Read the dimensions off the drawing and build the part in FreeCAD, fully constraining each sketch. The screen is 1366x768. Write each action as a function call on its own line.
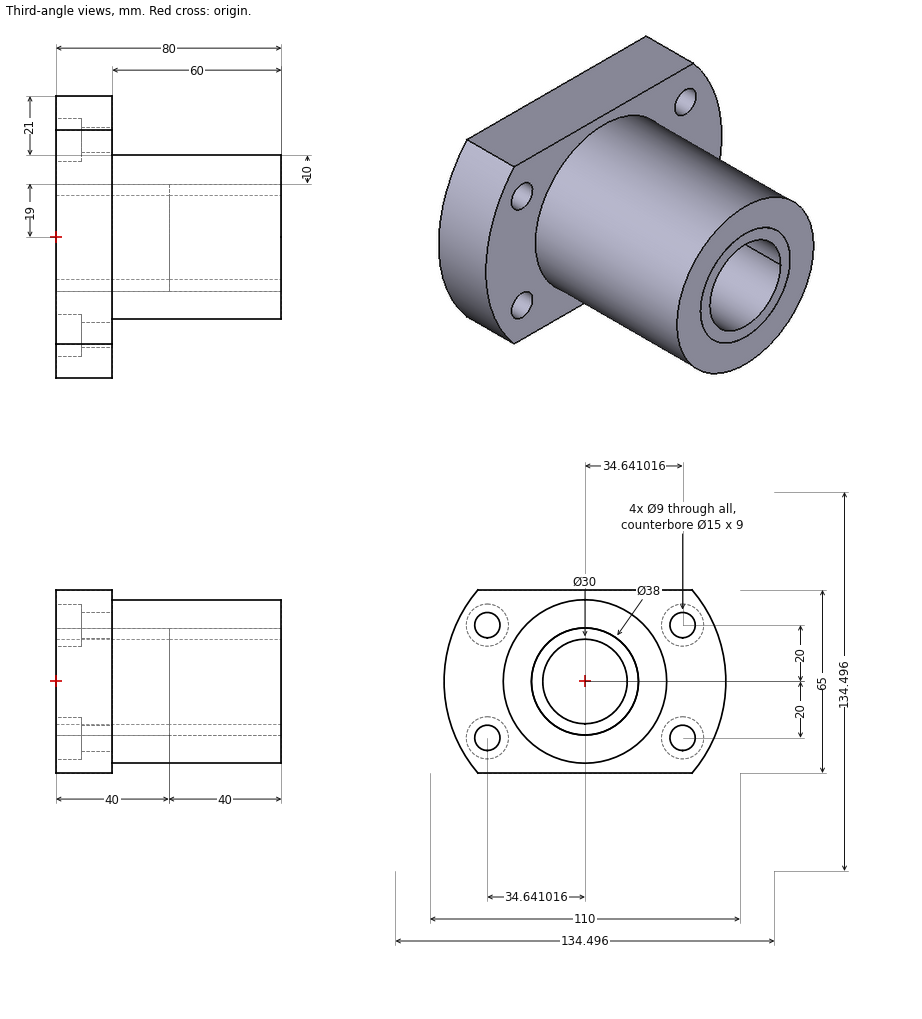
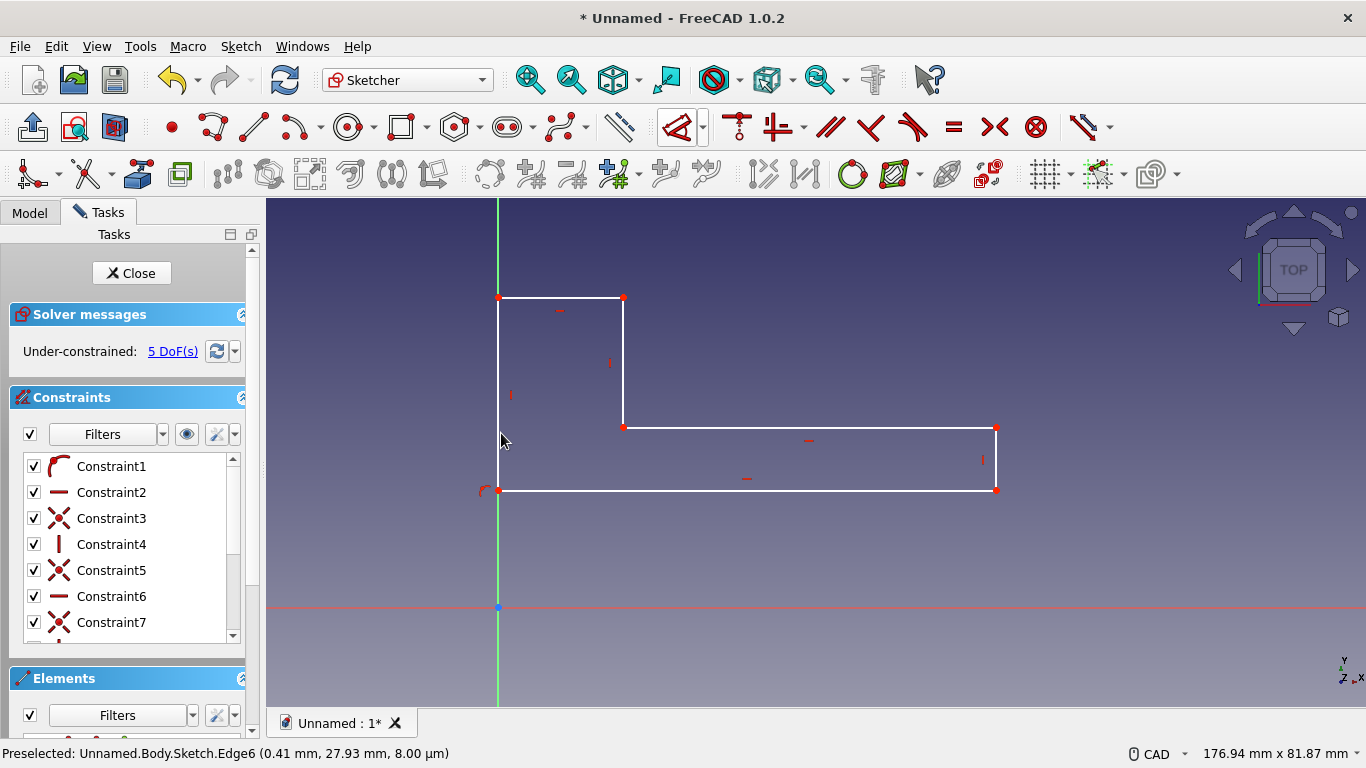
key(d)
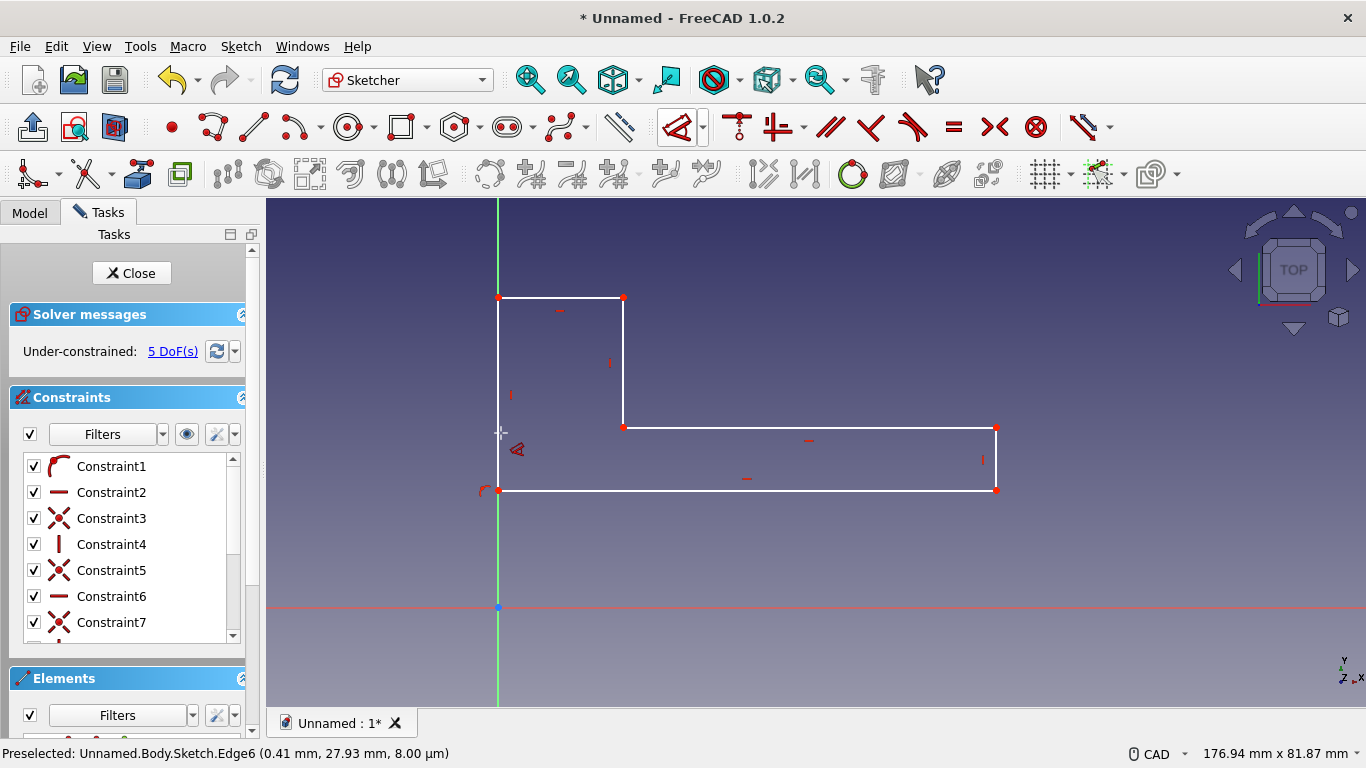
click(648, 491)
click(747, 525)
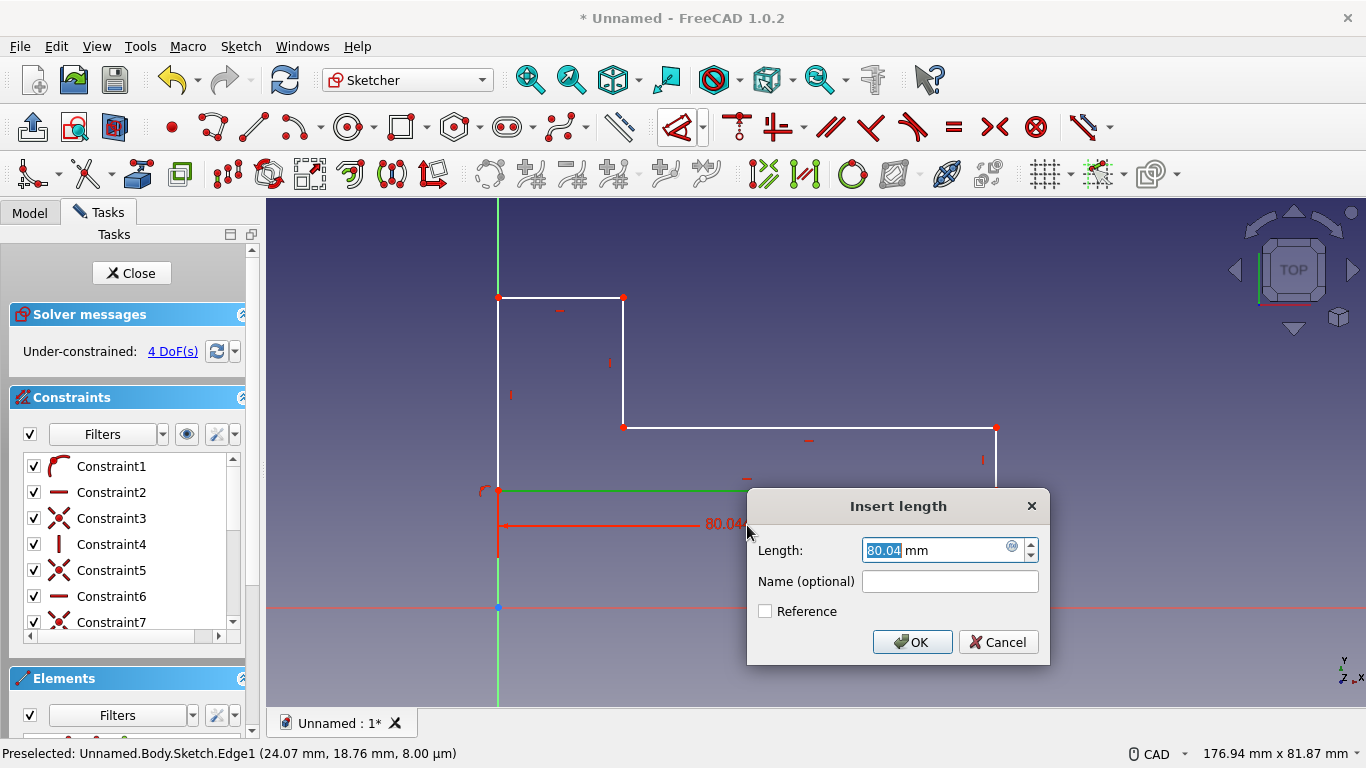
text(80)
key(Return)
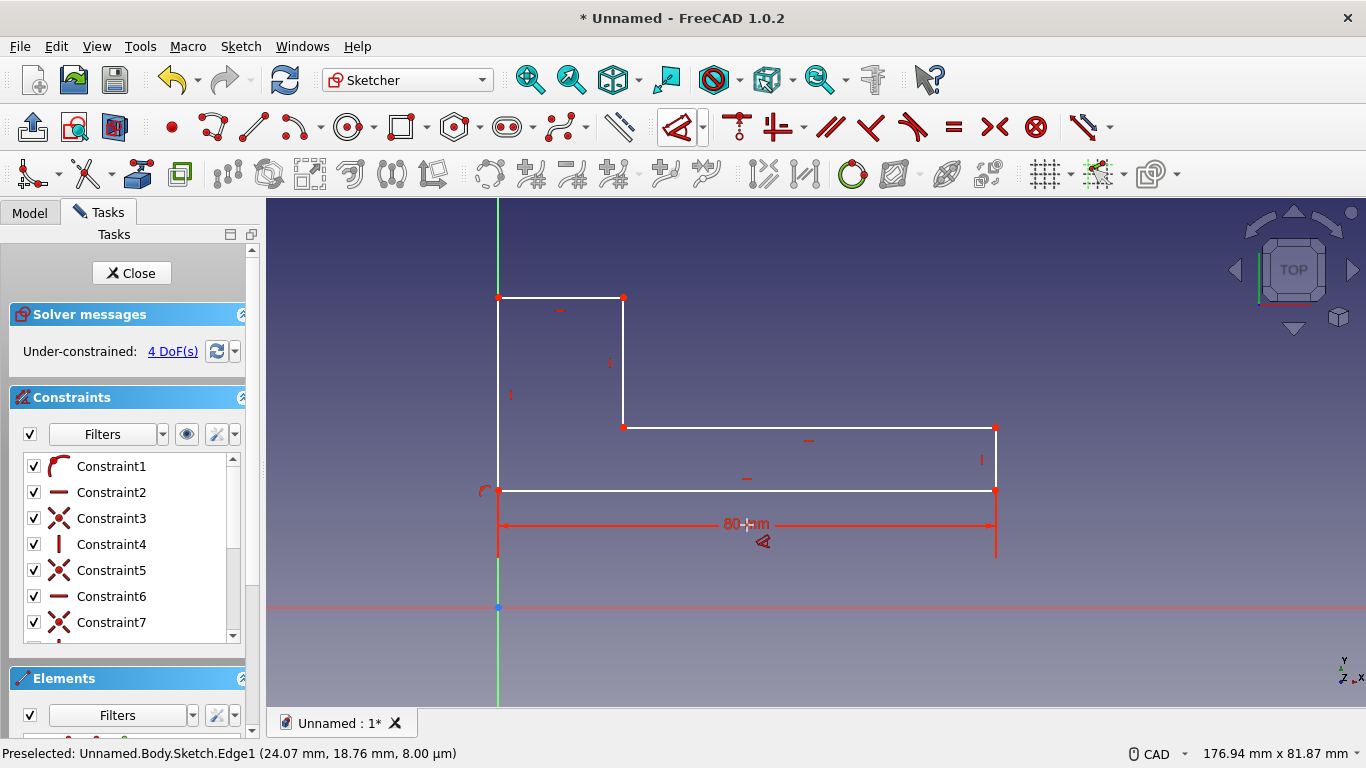
click(996, 472)
click(1030, 459)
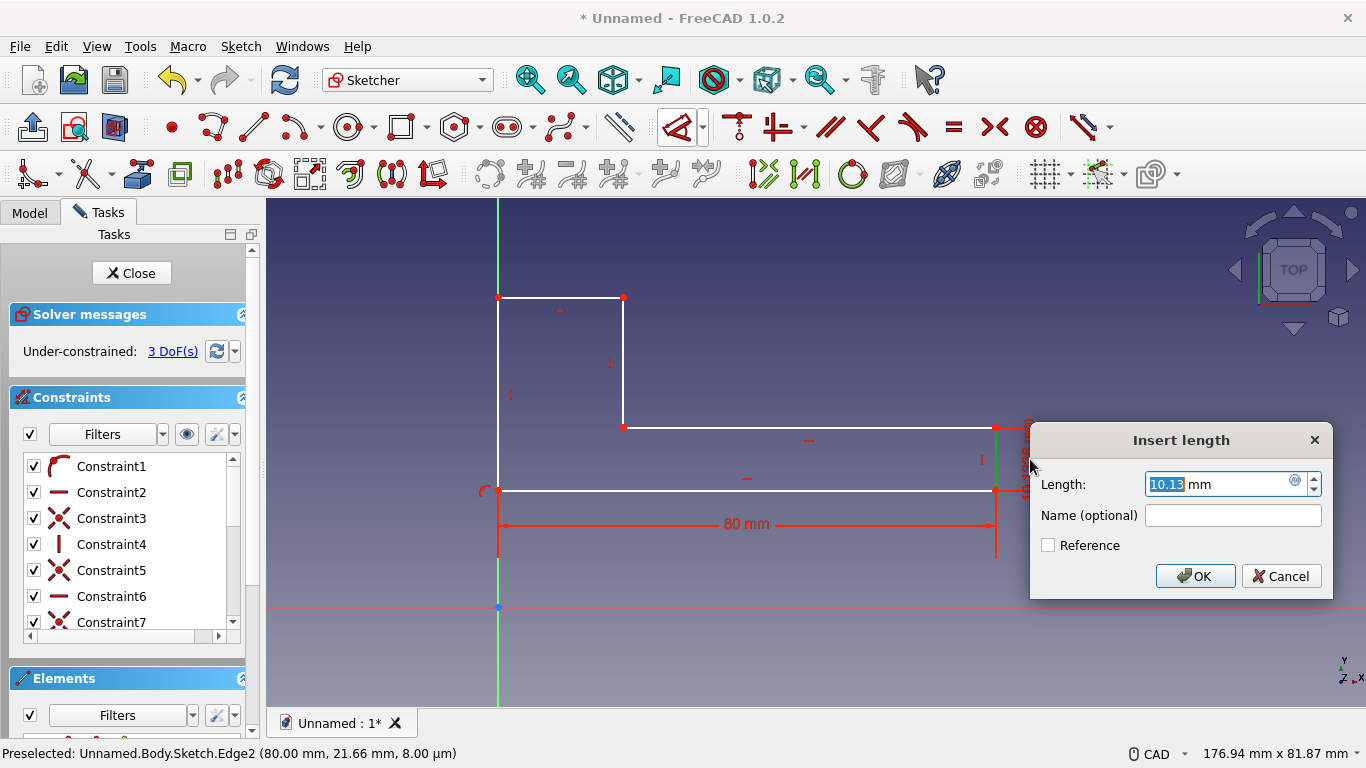
text(10)
key(Return)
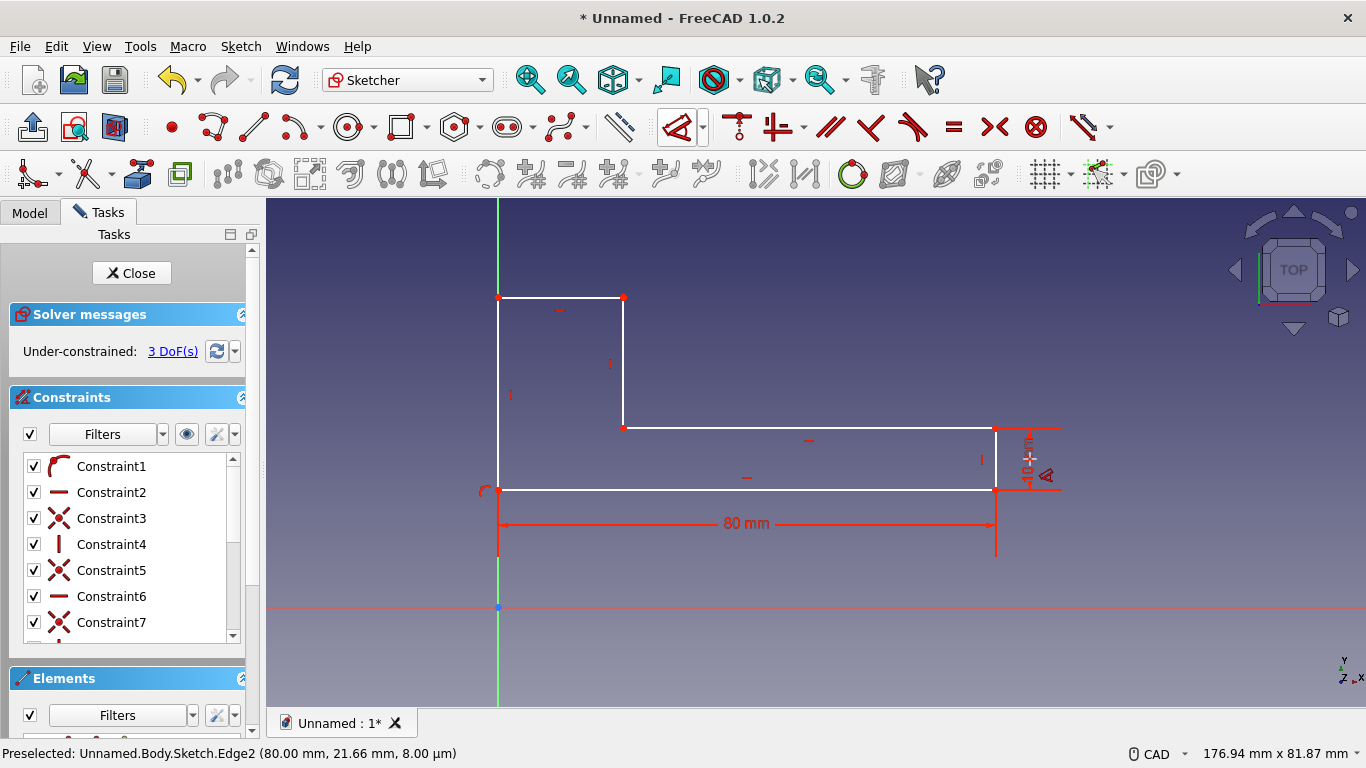
click(884, 428)
click(809, 394)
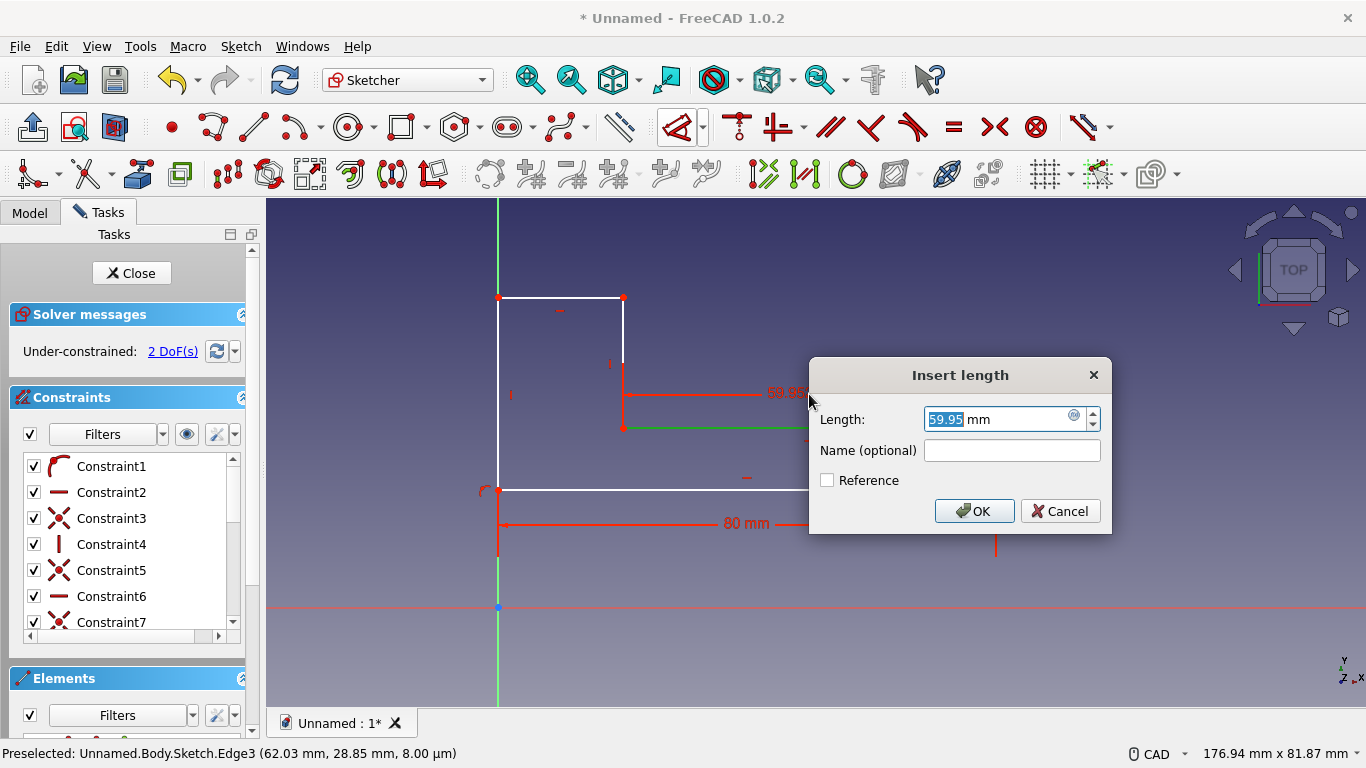
text(60)
key(Return)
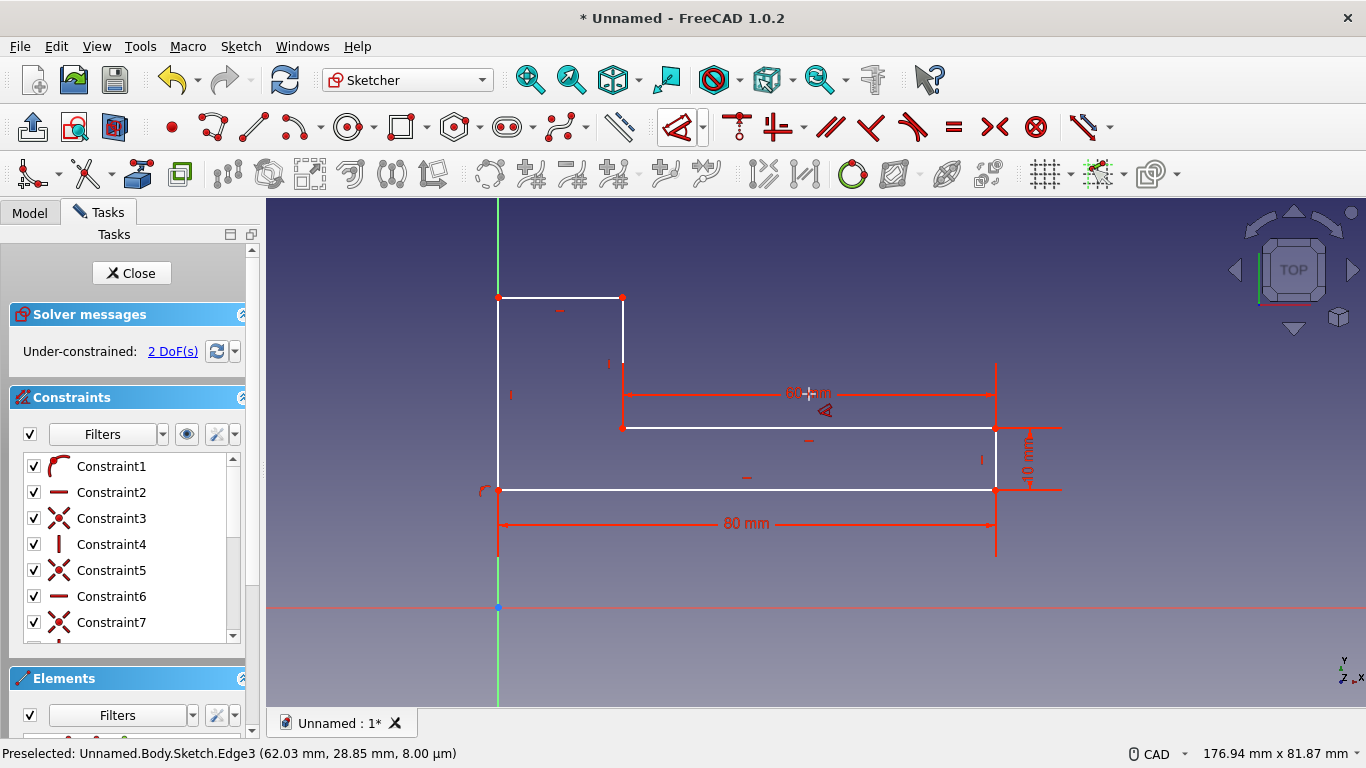
click(623, 389)
click(589, 363)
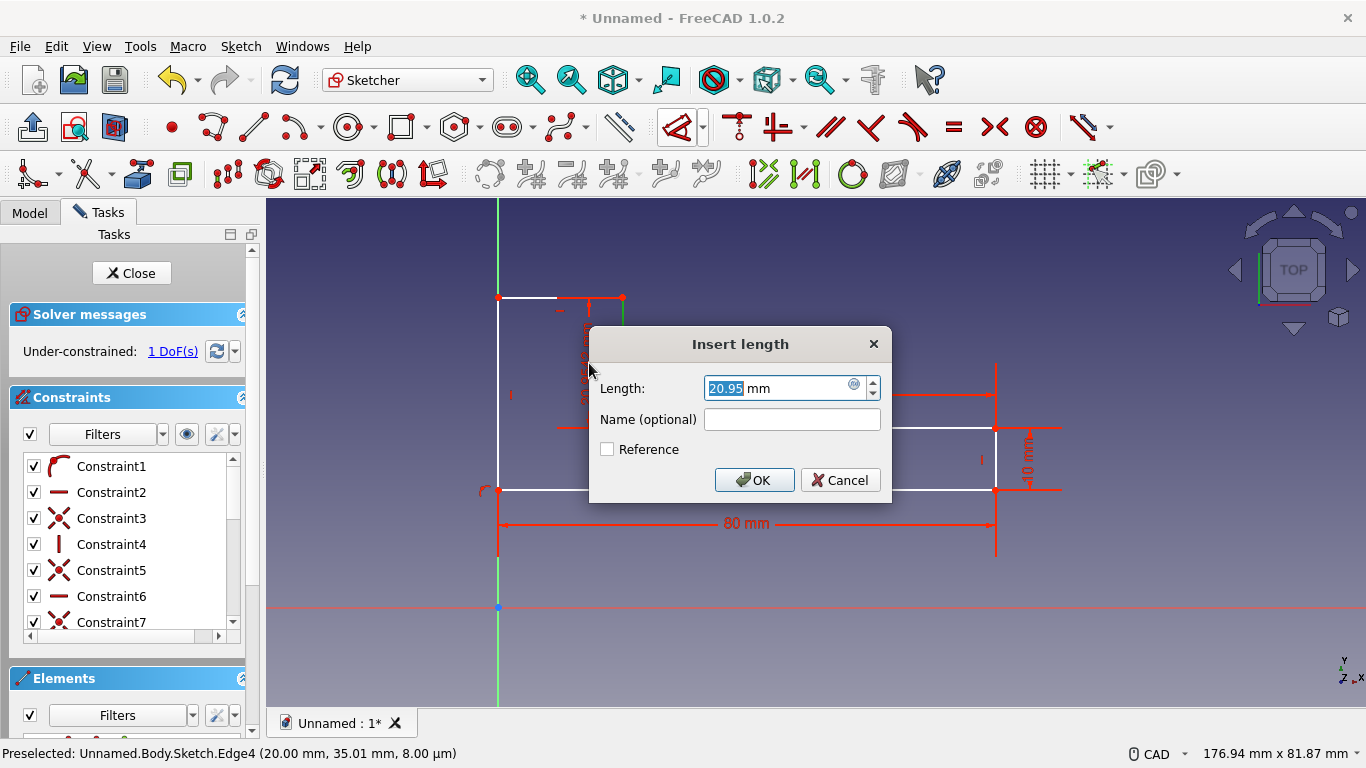
text(21)
key(Return)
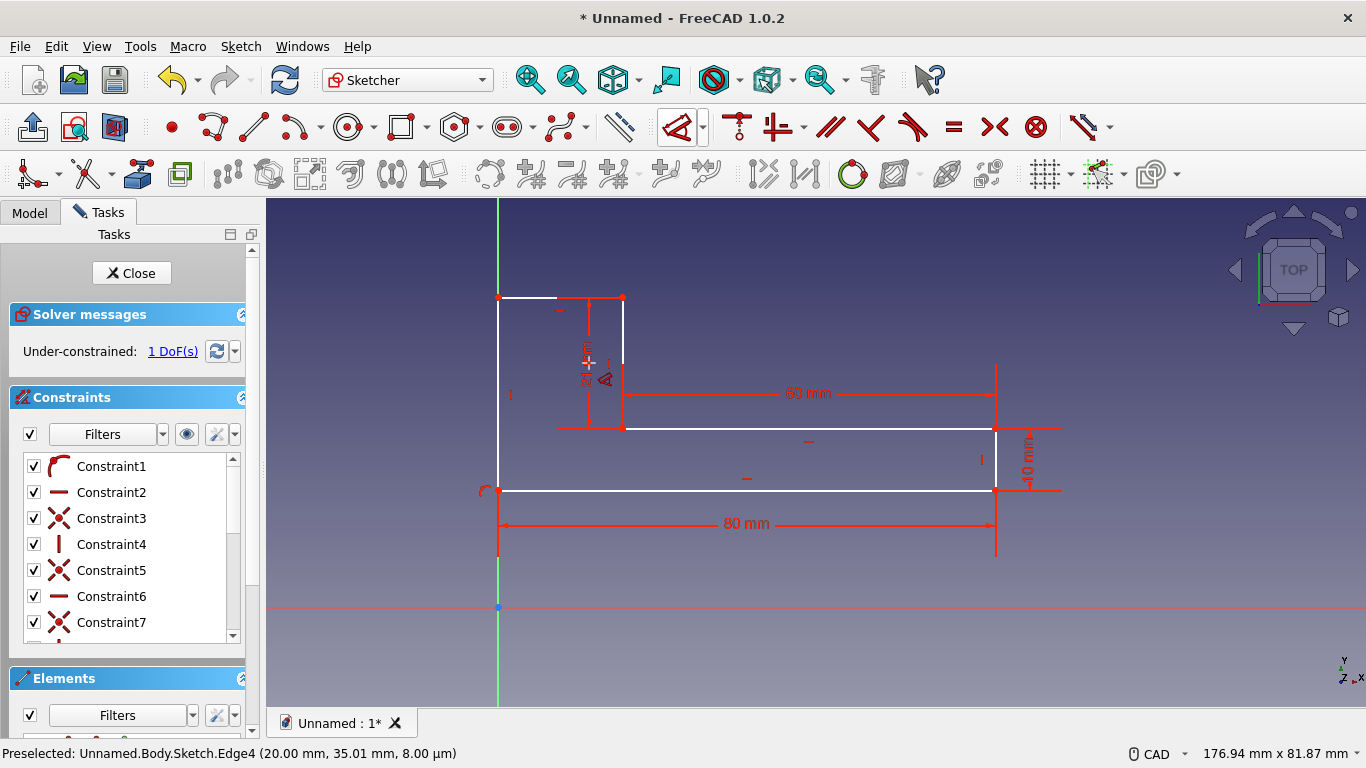
click(498, 491)
click(464, 549)